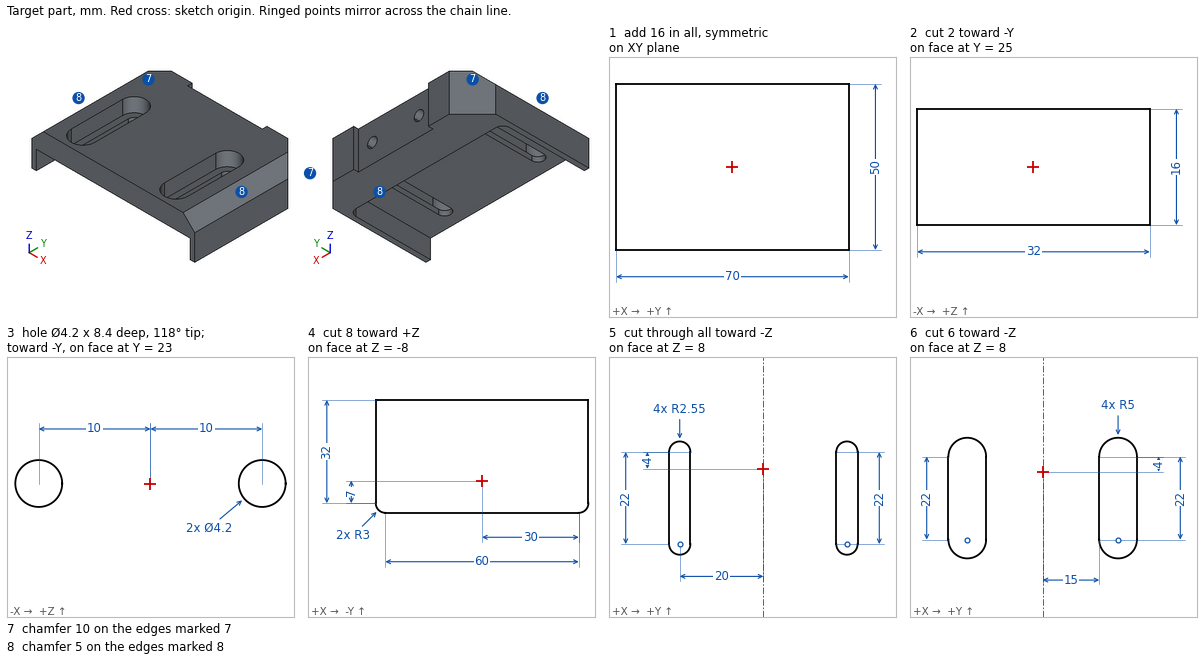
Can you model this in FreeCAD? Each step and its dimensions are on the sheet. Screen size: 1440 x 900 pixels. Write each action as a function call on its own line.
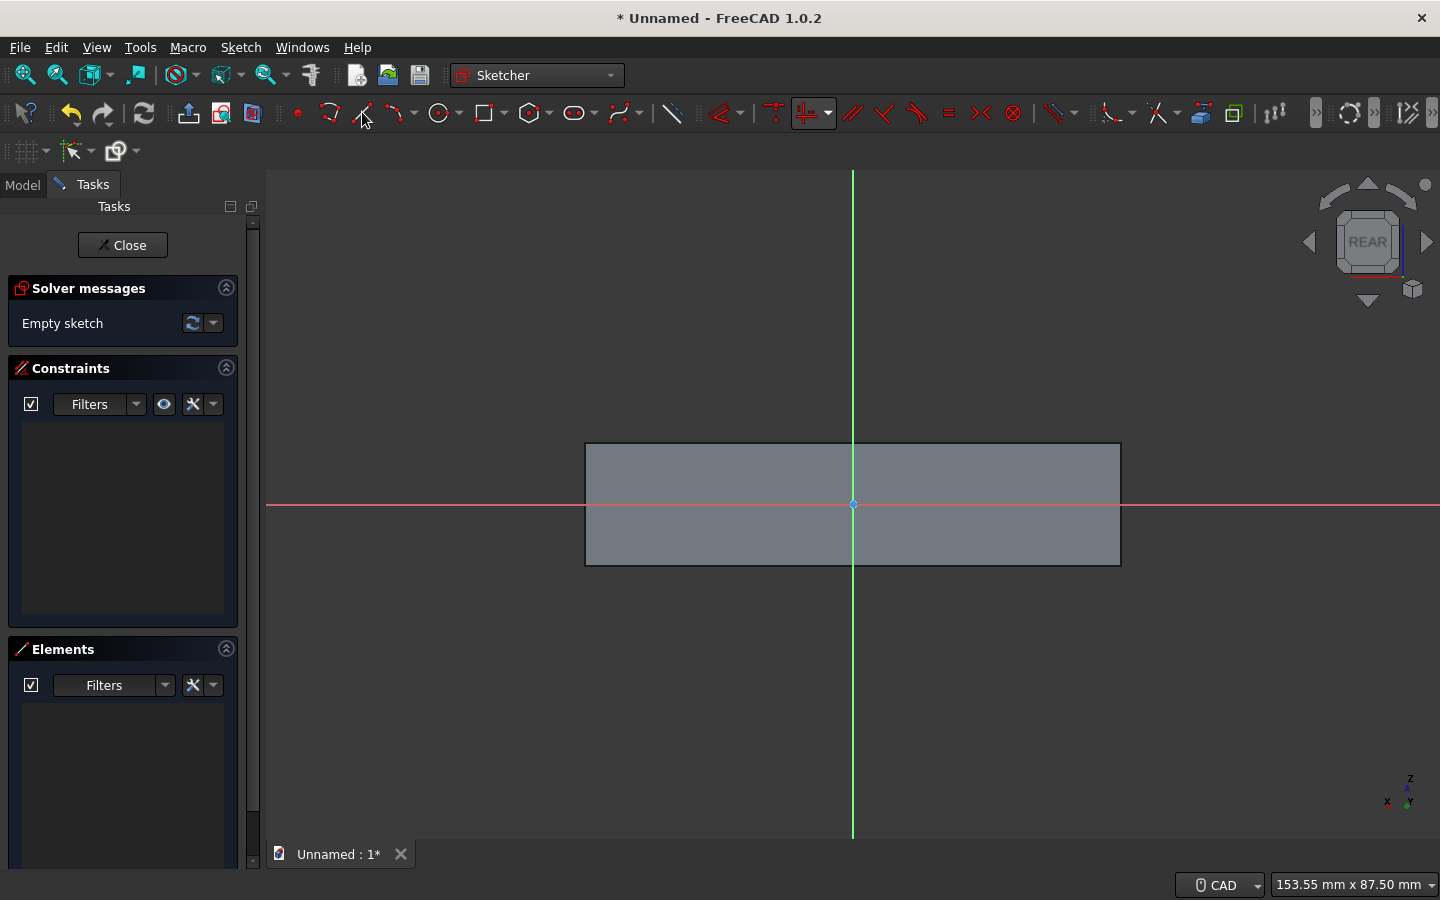
scroll(893, 504, up, 5)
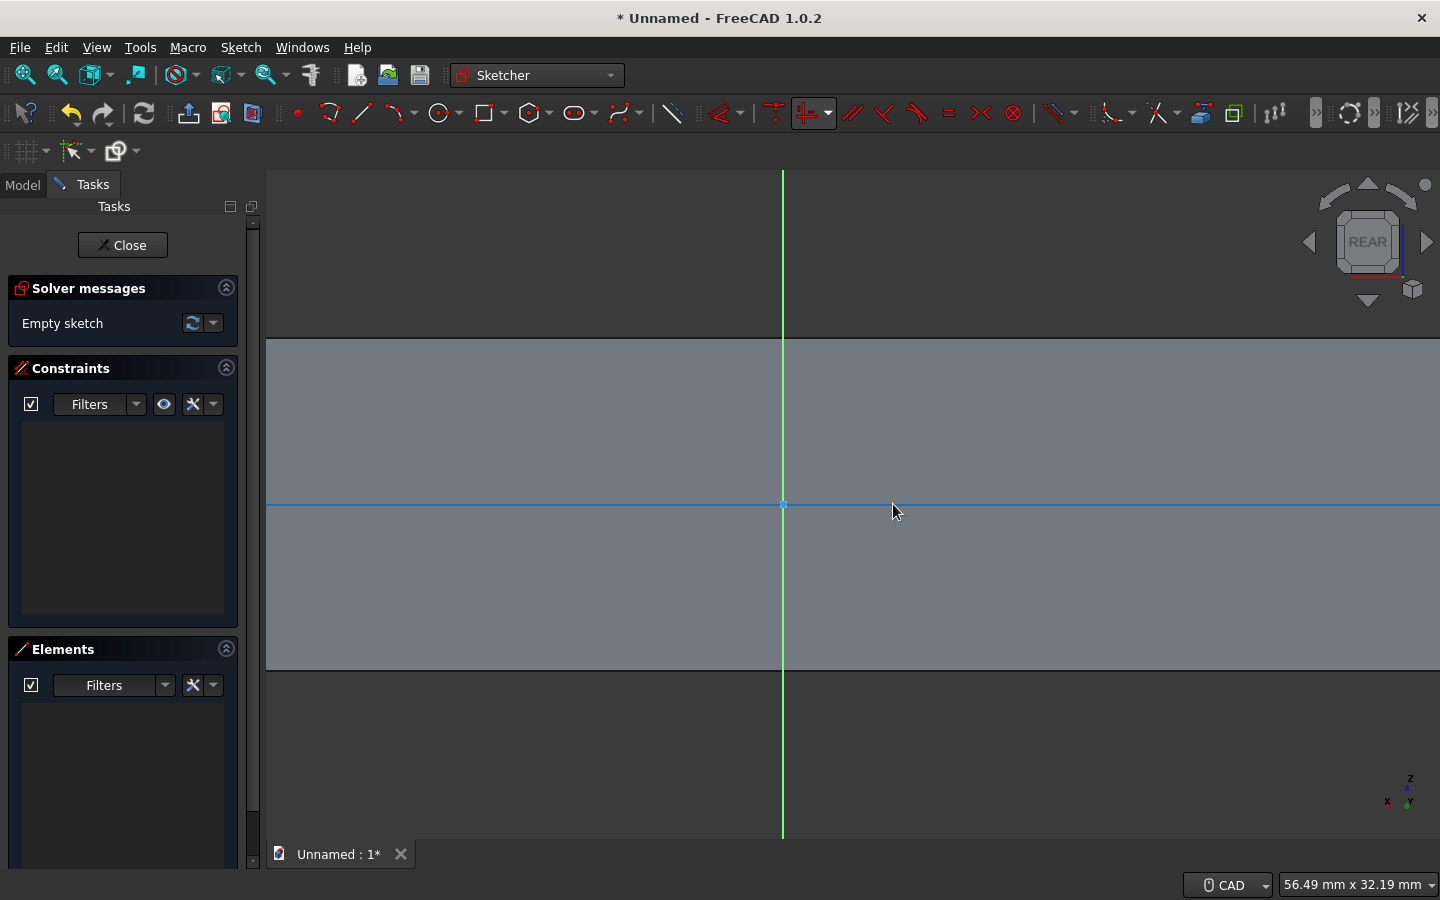
key(g)
key(v)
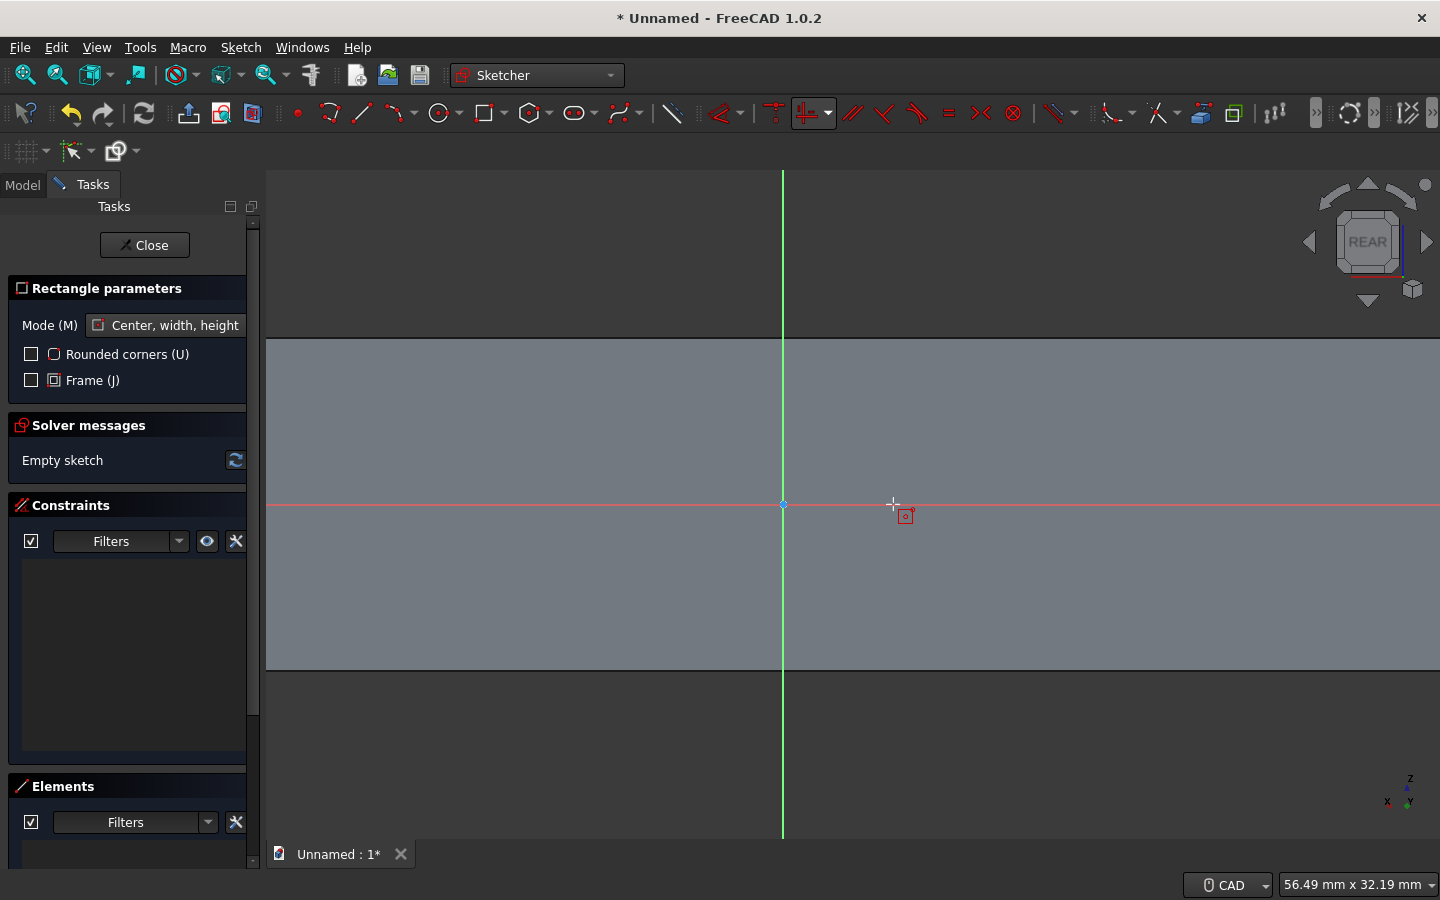
click(783, 504)
move(1116, 338)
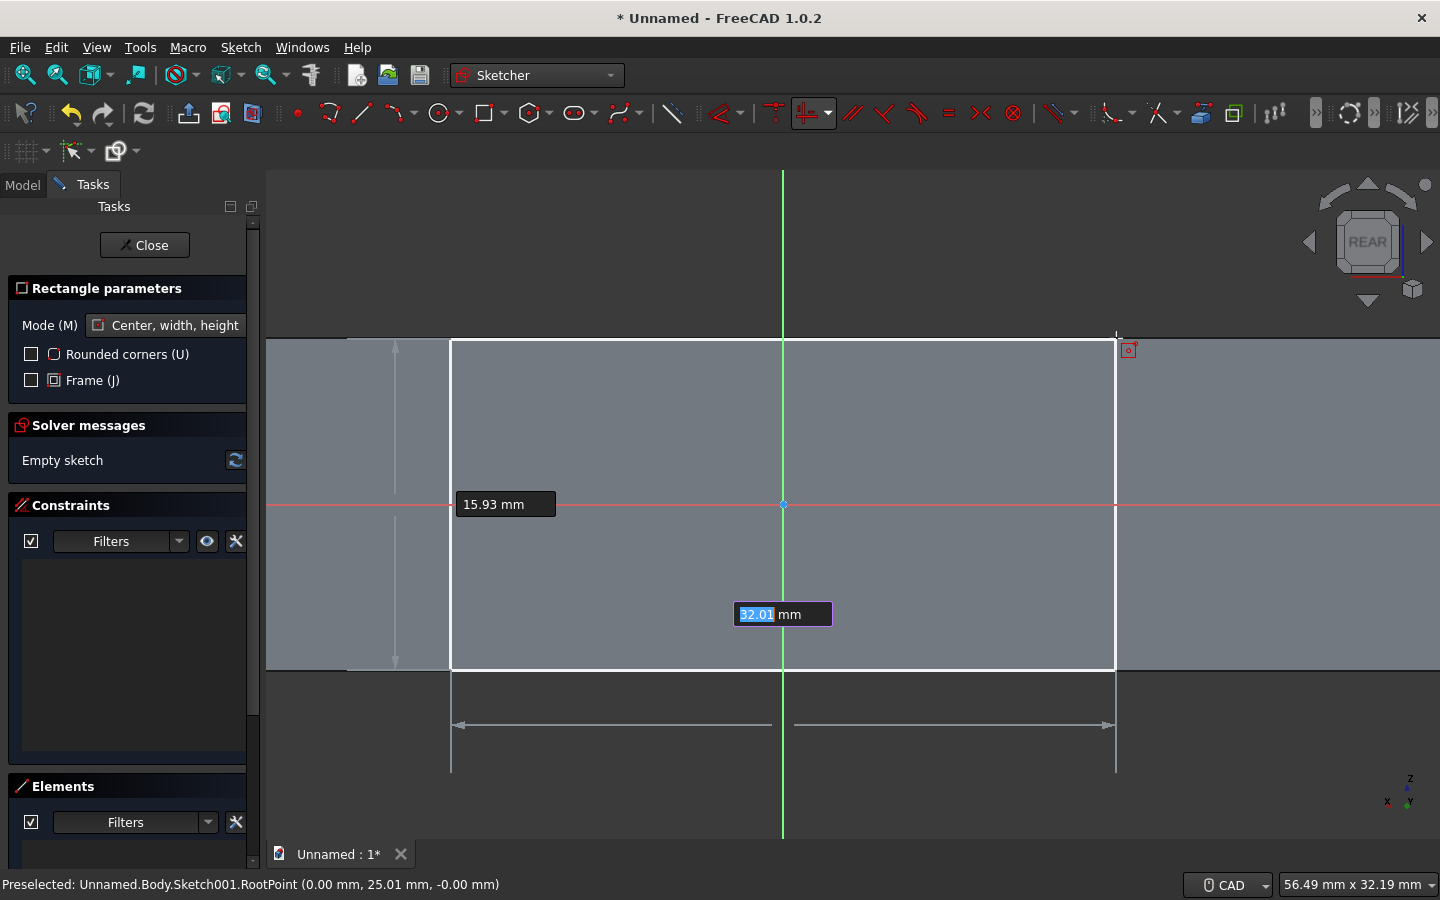
text(32)
key(Tab)
text(16)
key(Return)
key(Escape)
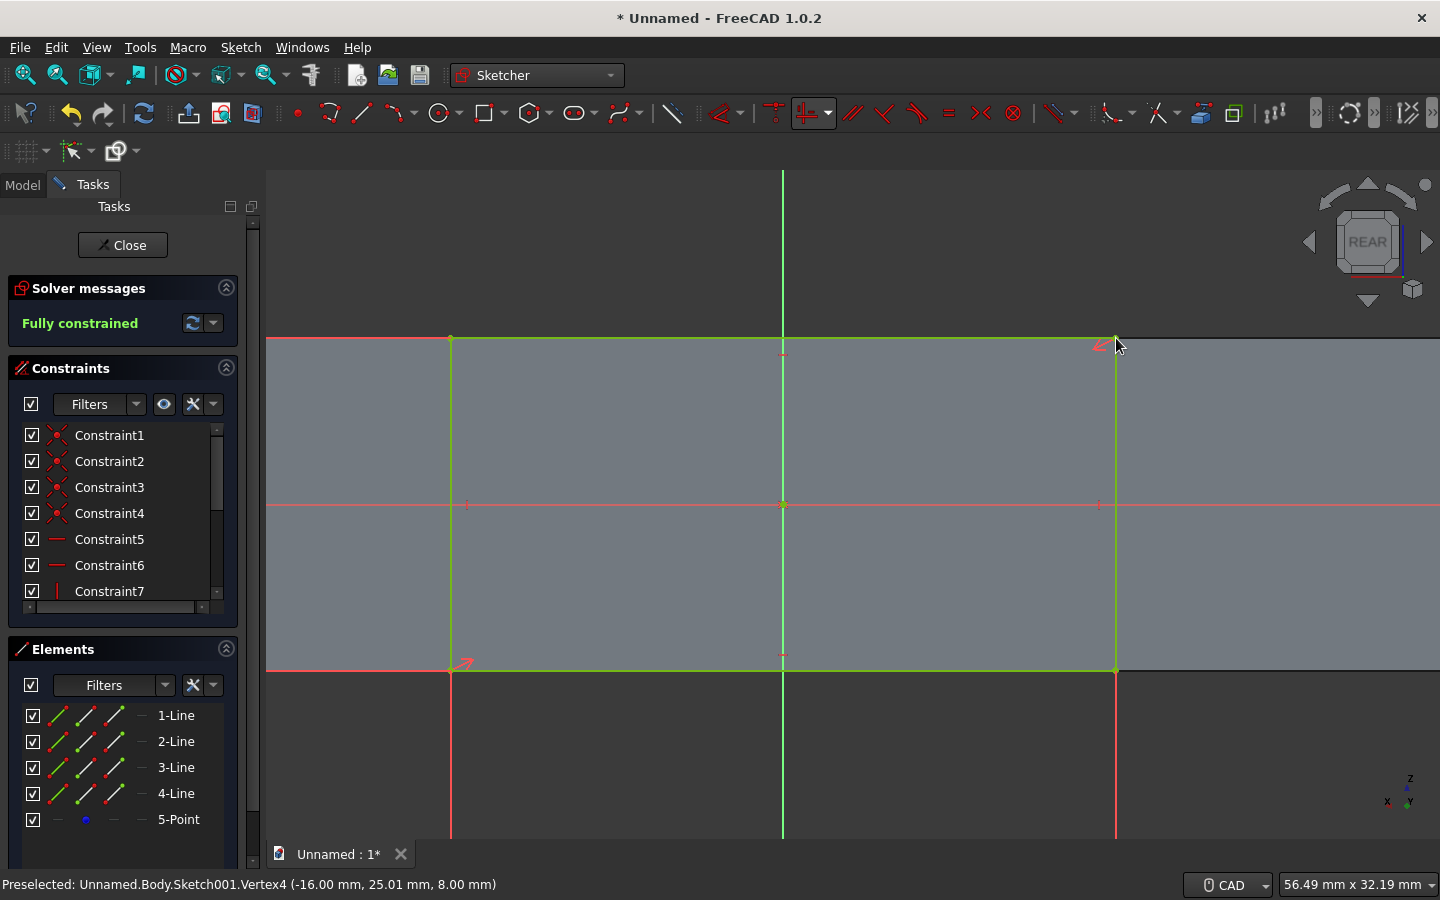
click(123, 245)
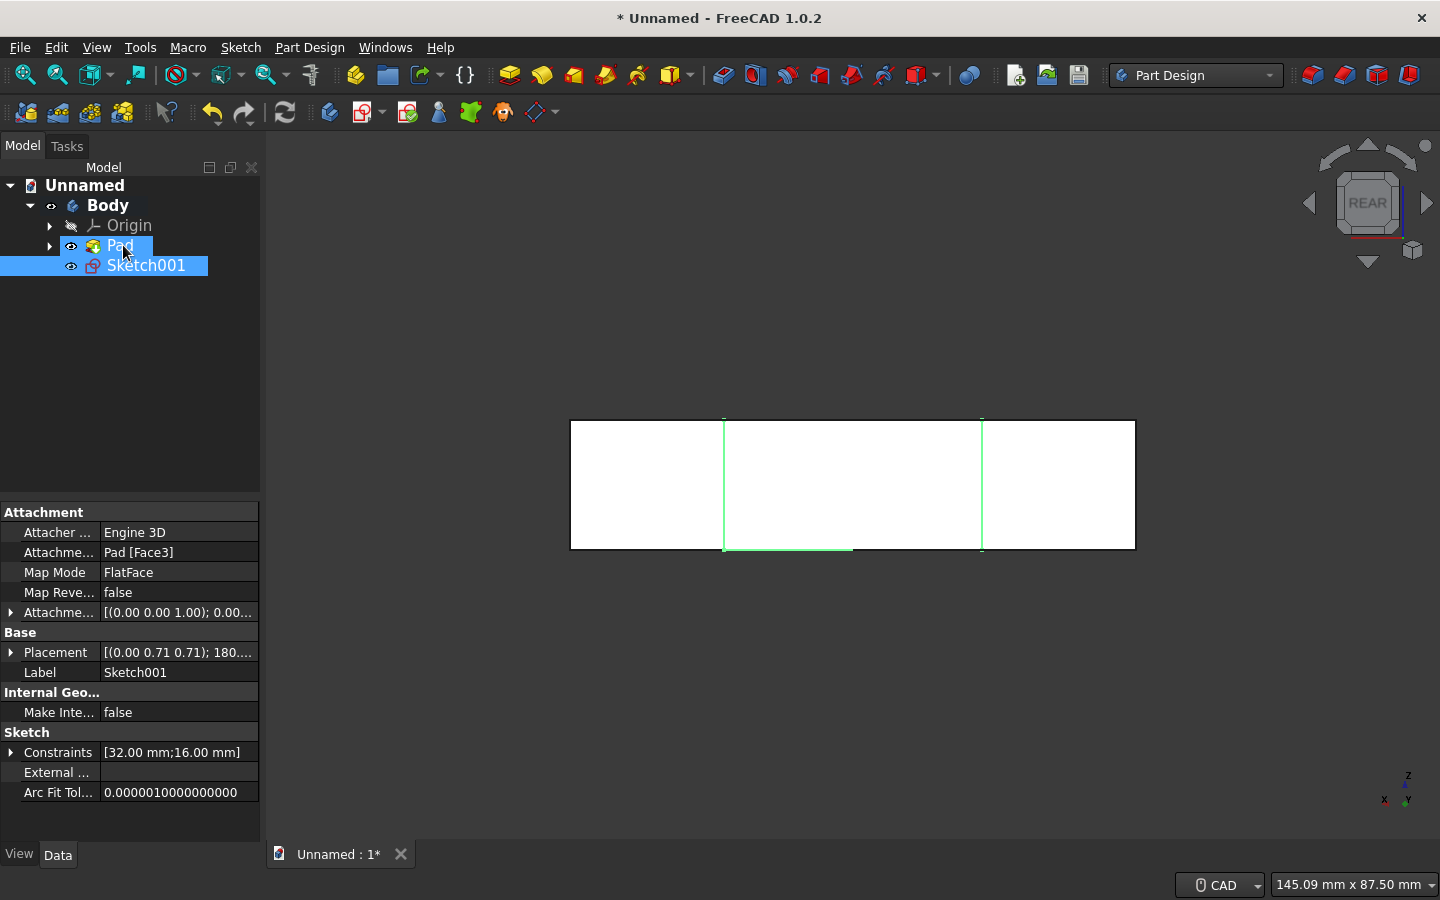
click(724, 76)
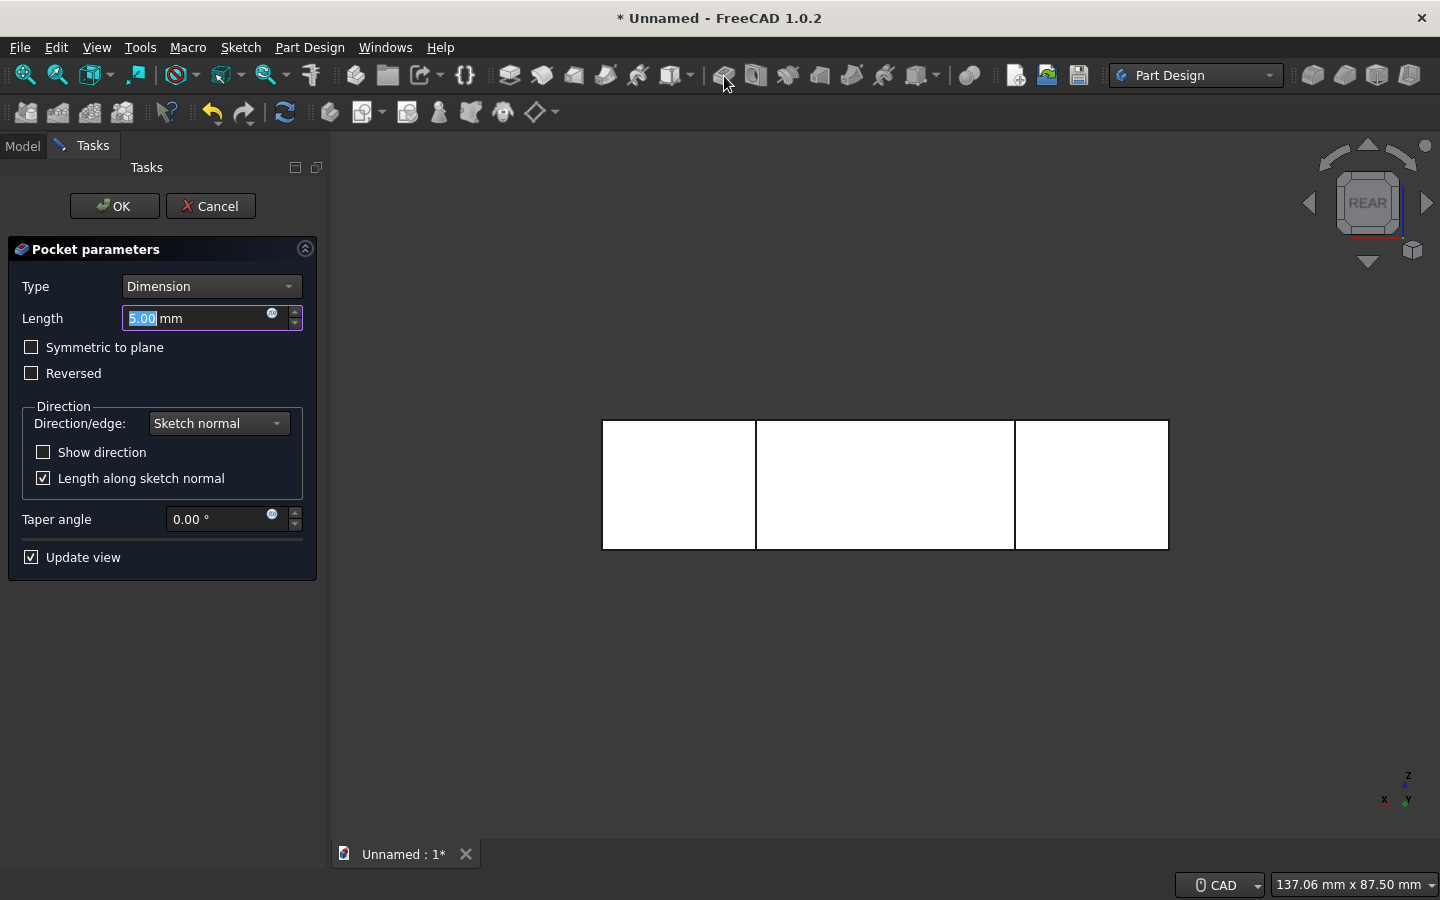
text(2)
key(Tab)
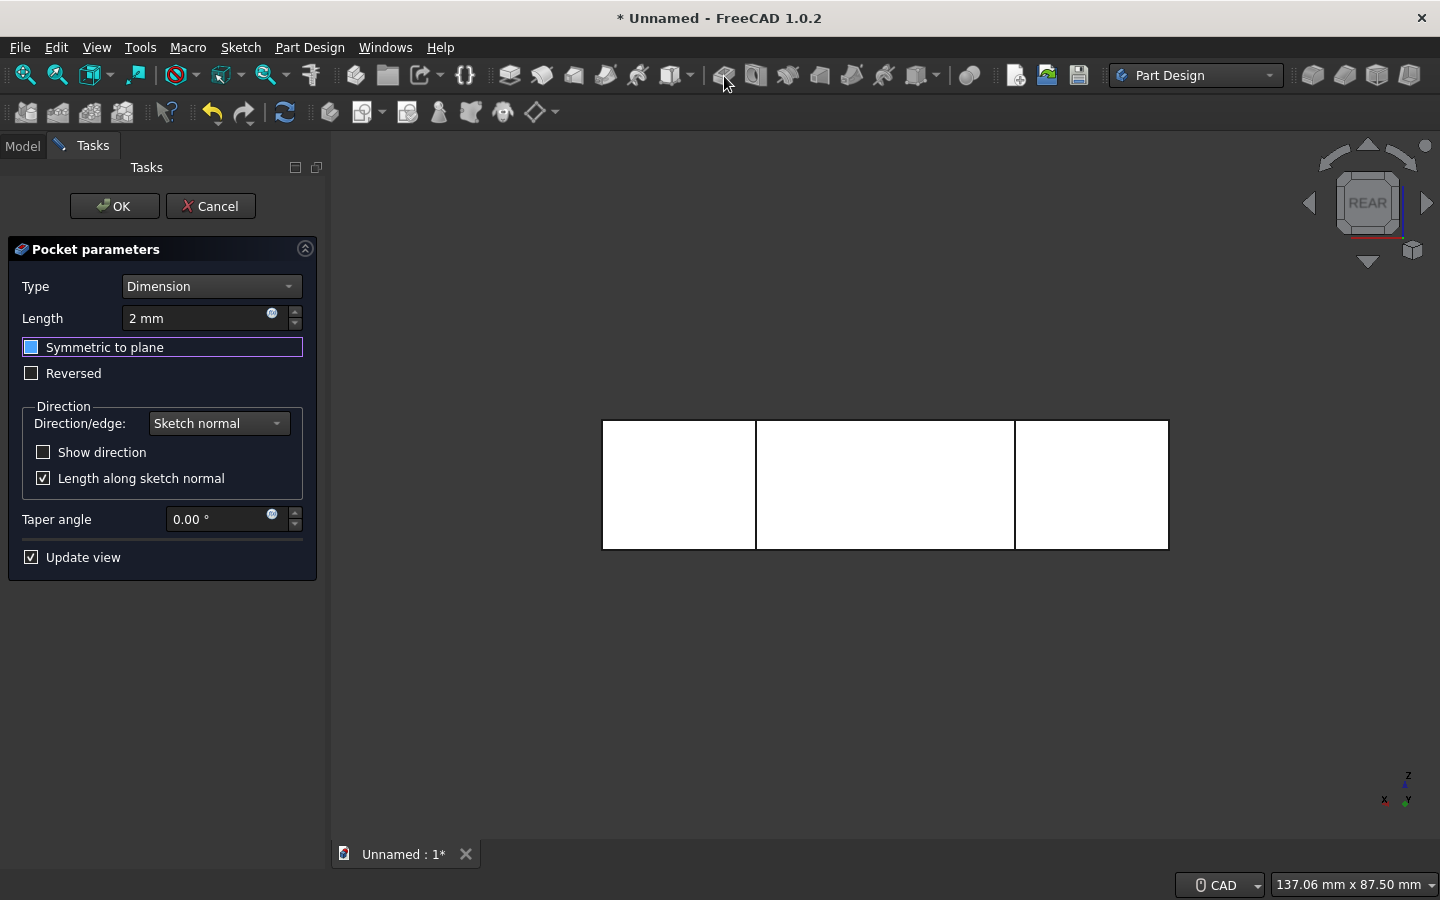
click(115, 206)